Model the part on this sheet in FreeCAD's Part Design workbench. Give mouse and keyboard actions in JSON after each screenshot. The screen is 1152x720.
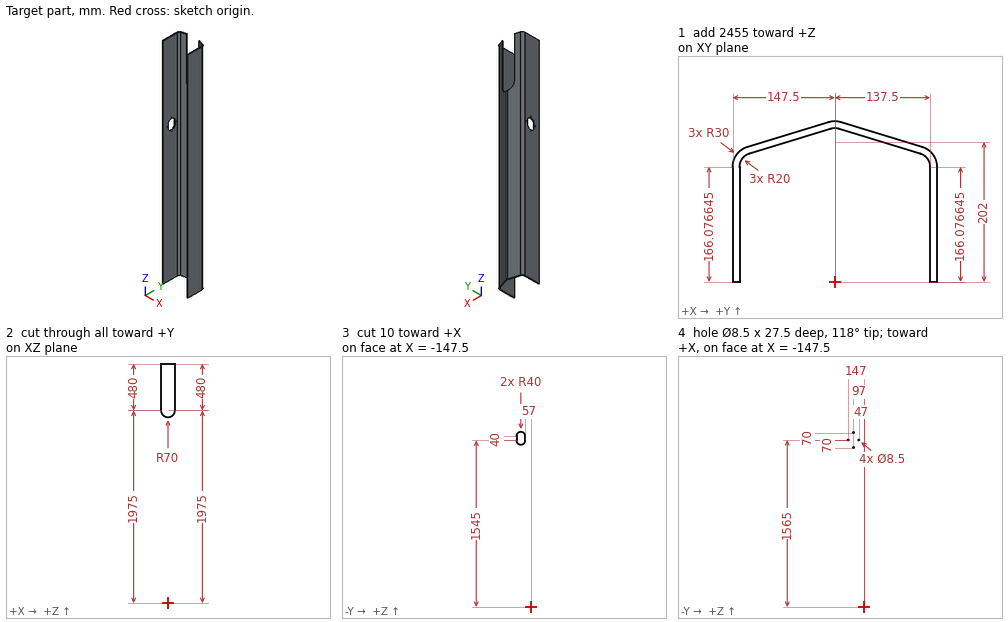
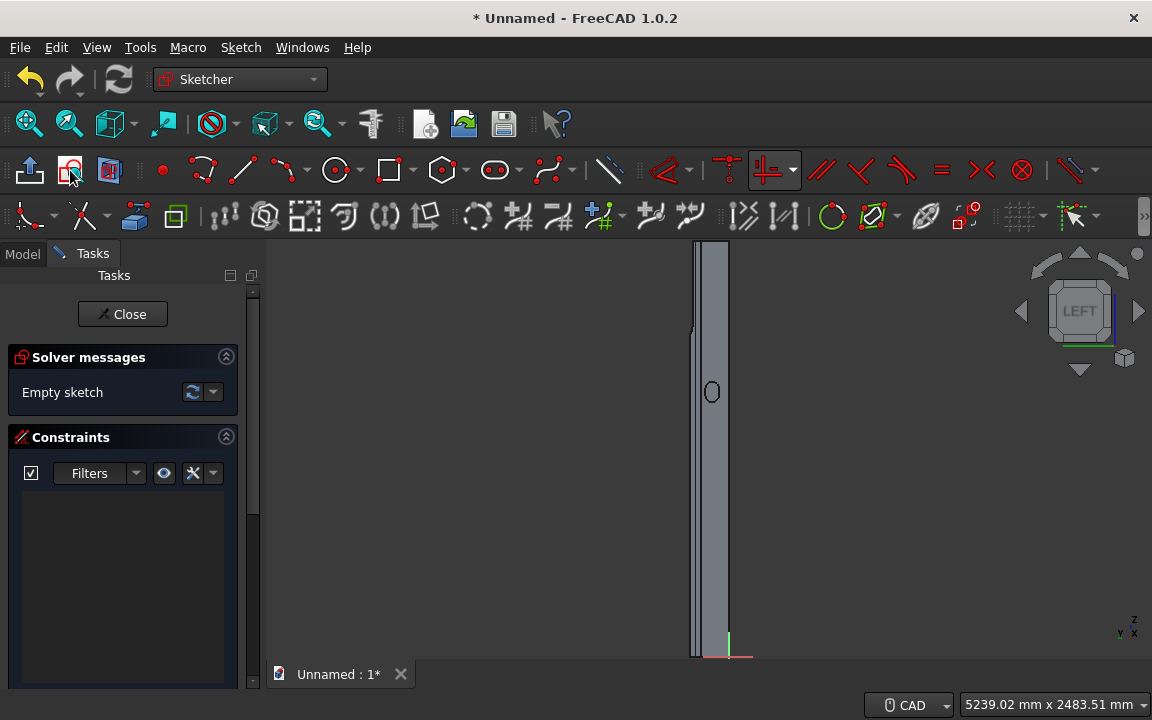
{"action": "scroll", "coordinate": [719, 386], "scroll_direction": "up", "scroll_amount": 12}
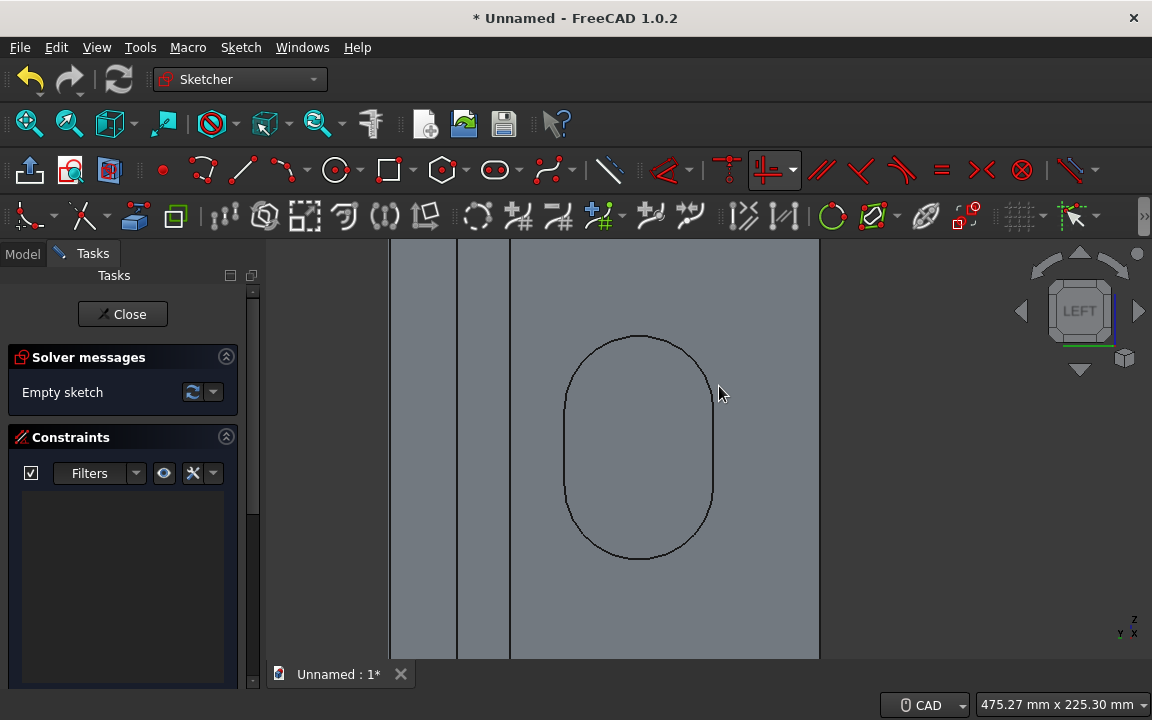
{"action": "left_click", "coordinate": [336, 170]}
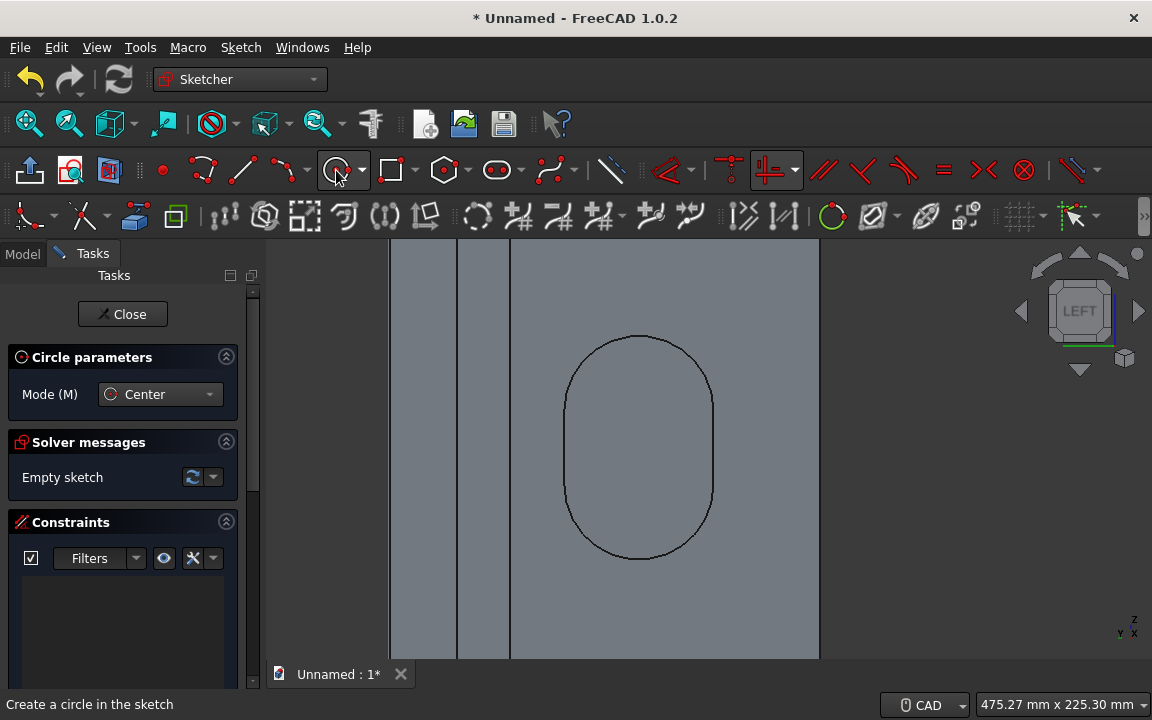
{"action": "scroll", "coordinate": [546, 448], "scroll_direction": "up", "scroll_amount": 6}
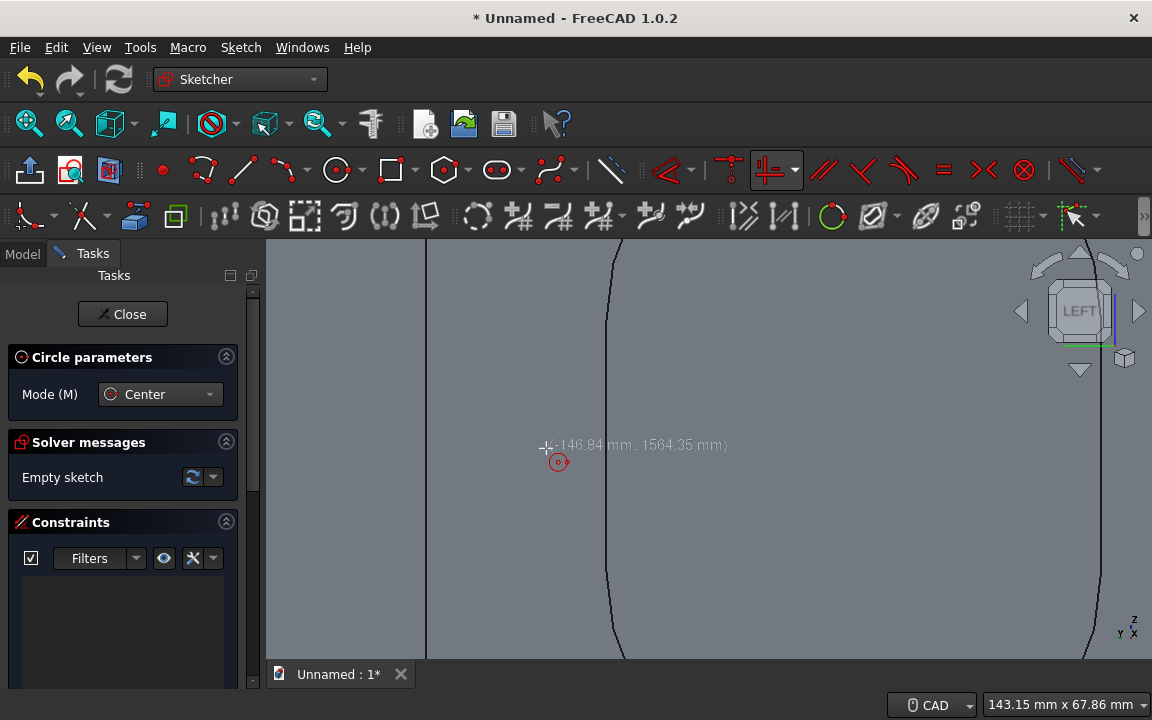
{"action": "left_click", "coordinate": [544, 446]}
{"action": "left_click", "coordinate": [563, 428]}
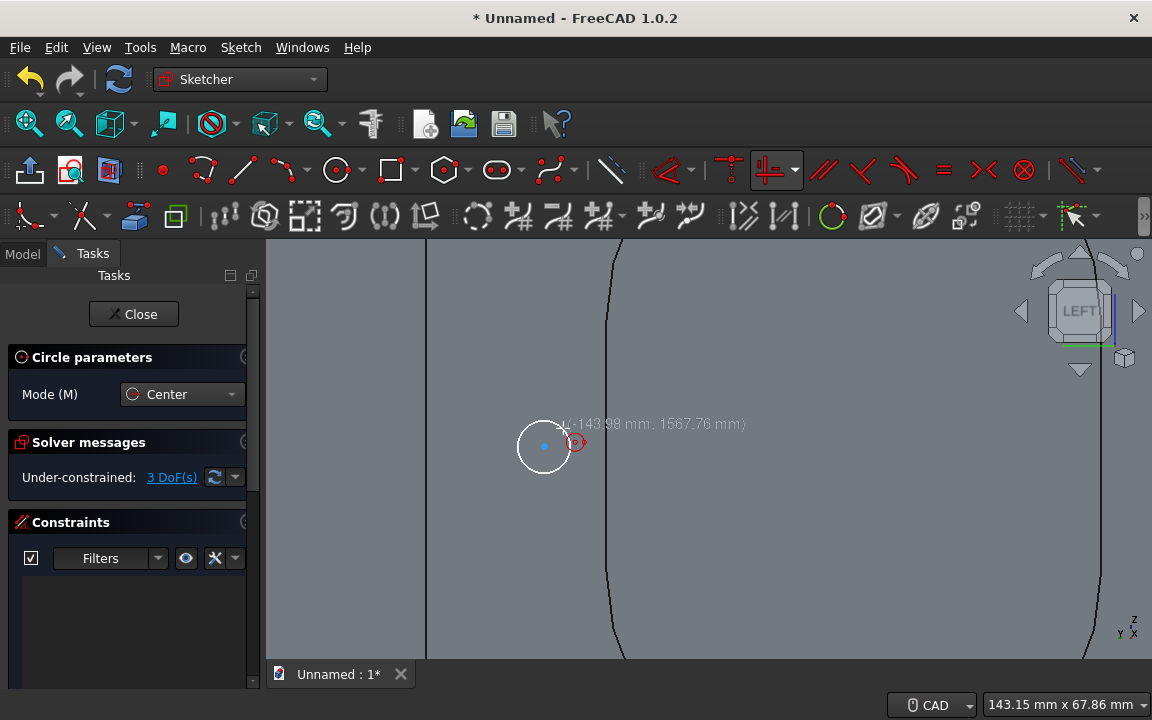
{"action": "scroll", "coordinate": [549, 450], "scroll_direction": "down", "scroll_amount": 6}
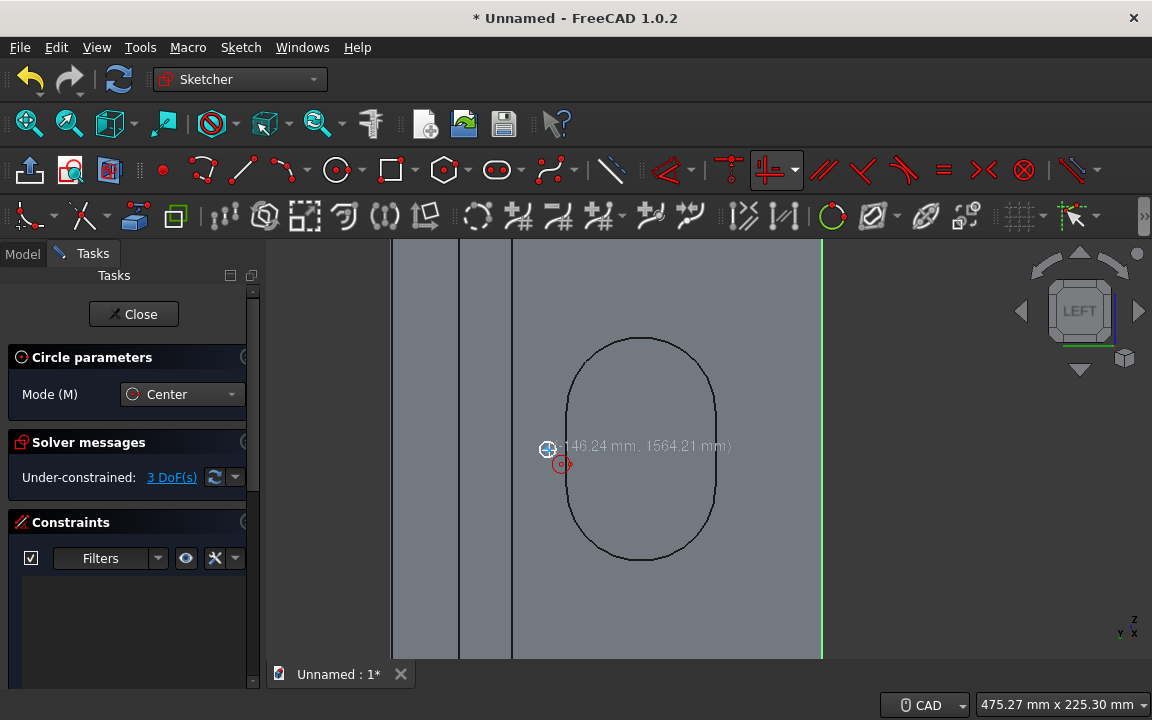
{"action": "scroll", "coordinate": [734, 449], "scroll_direction": "up", "scroll_amount": 6}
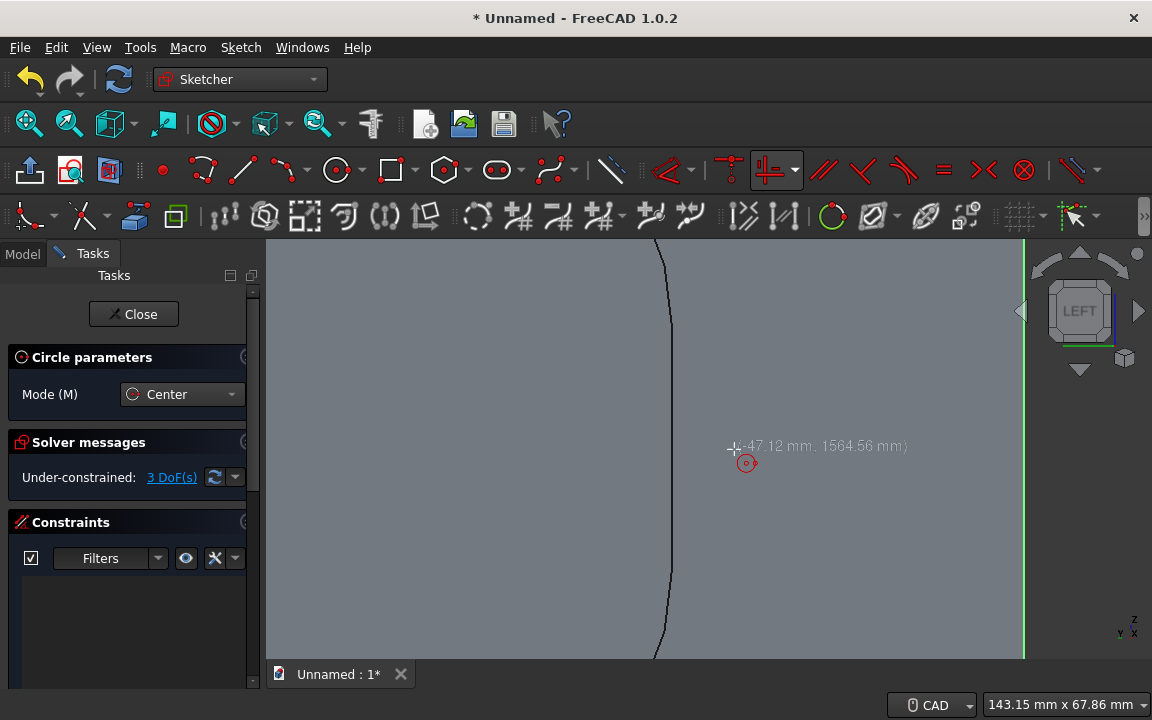
{"action": "left_click", "coordinate": [734, 448]}
{"action": "left_click", "coordinate": [752, 430]}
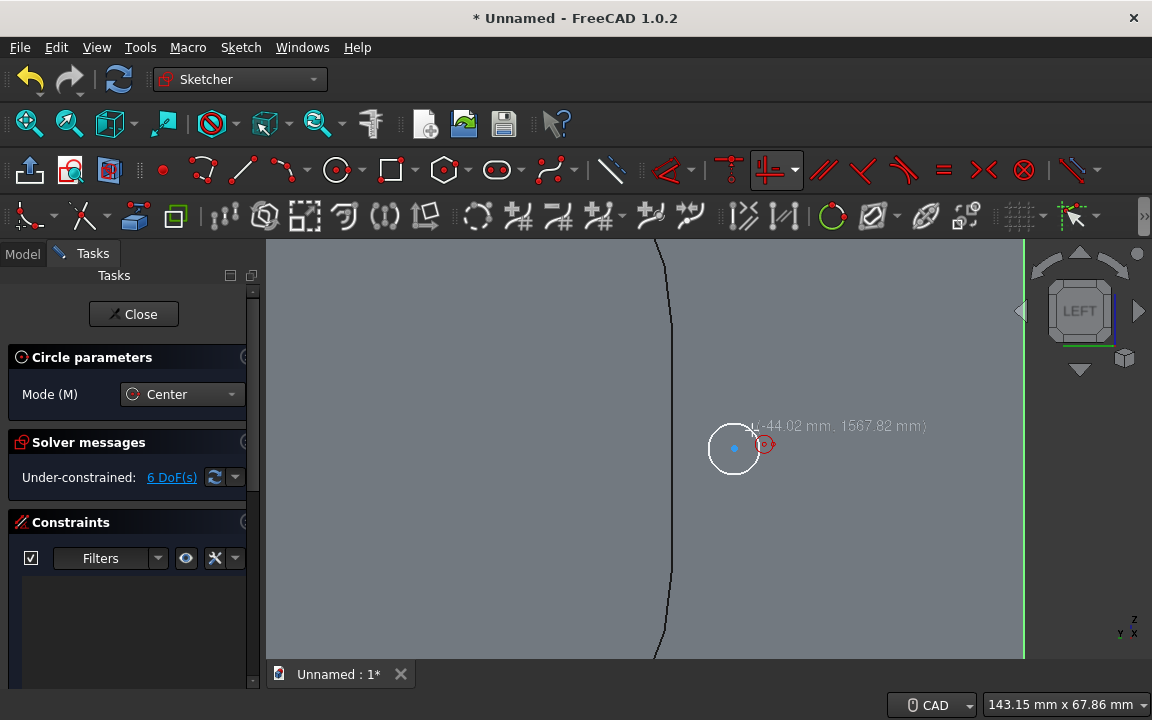
{"action": "scroll", "coordinate": [734, 449], "scroll_direction": "down", "scroll_amount": 6}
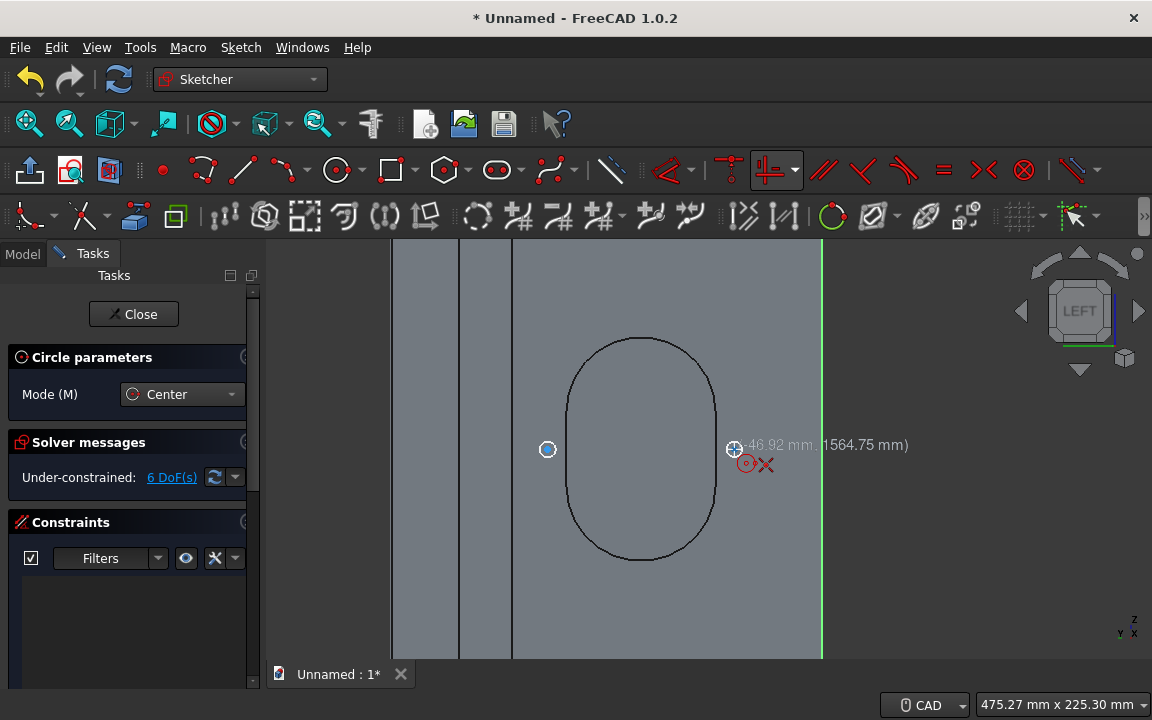
{"action": "scroll", "coordinate": [641, 580], "scroll_direction": "up", "scroll_amount": 6}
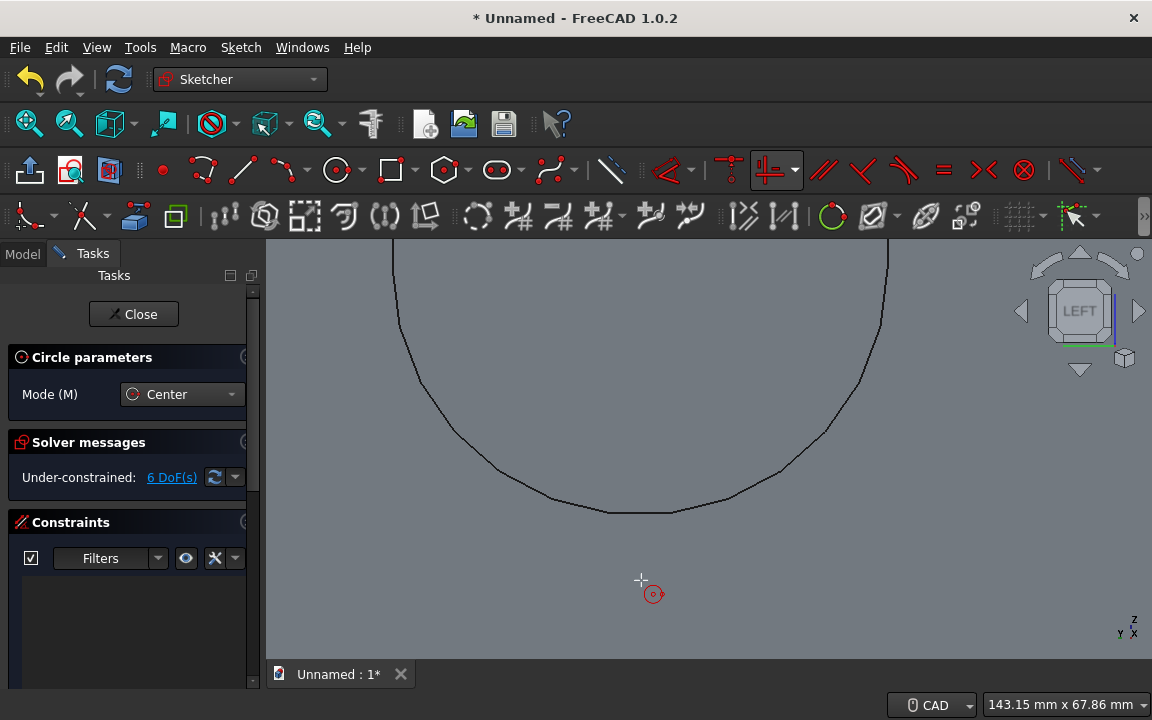
{"action": "left_click", "coordinate": [640, 577]}
{"action": "left_click", "coordinate": [659, 558]}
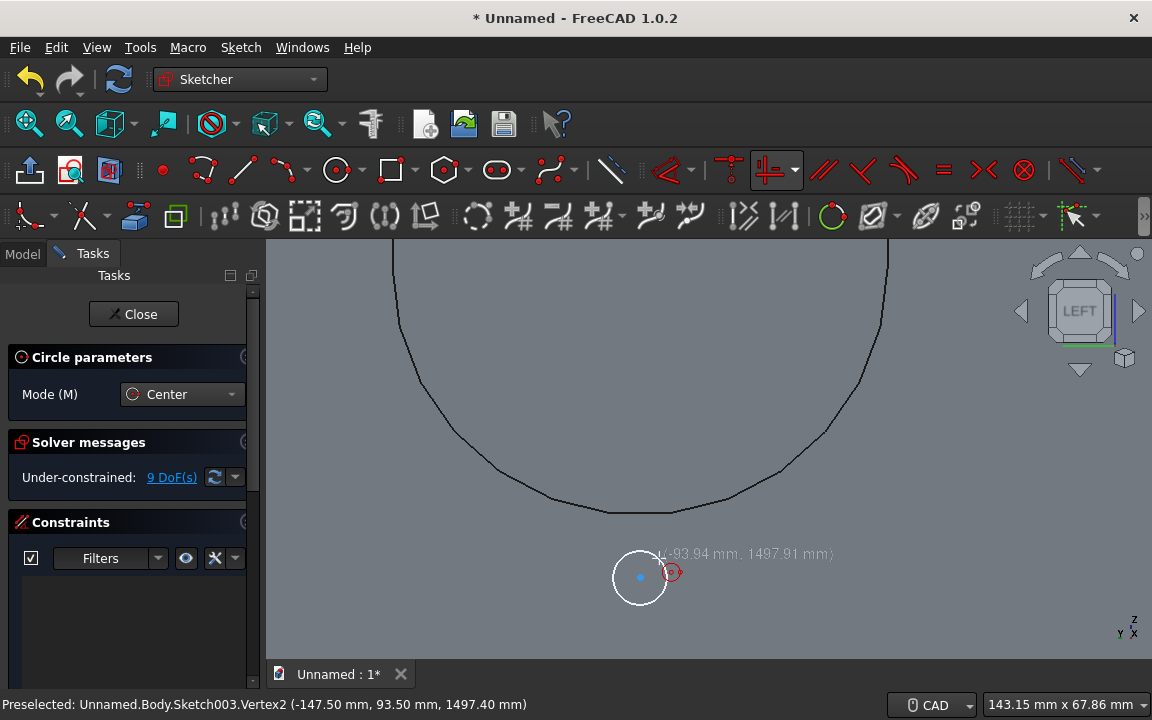
{"action": "scroll", "coordinate": [641, 581], "scroll_direction": "down", "scroll_amount": 6}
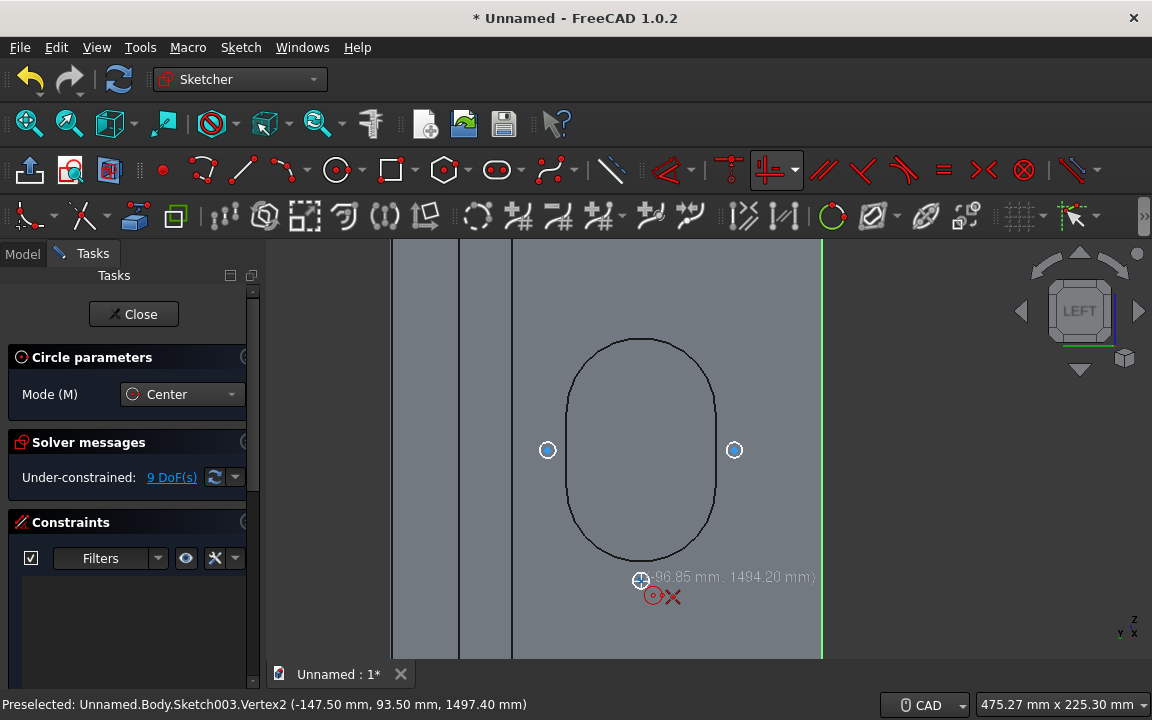
{"action": "scroll", "coordinate": [641, 319], "scroll_direction": "up", "scroll_amount": 6}